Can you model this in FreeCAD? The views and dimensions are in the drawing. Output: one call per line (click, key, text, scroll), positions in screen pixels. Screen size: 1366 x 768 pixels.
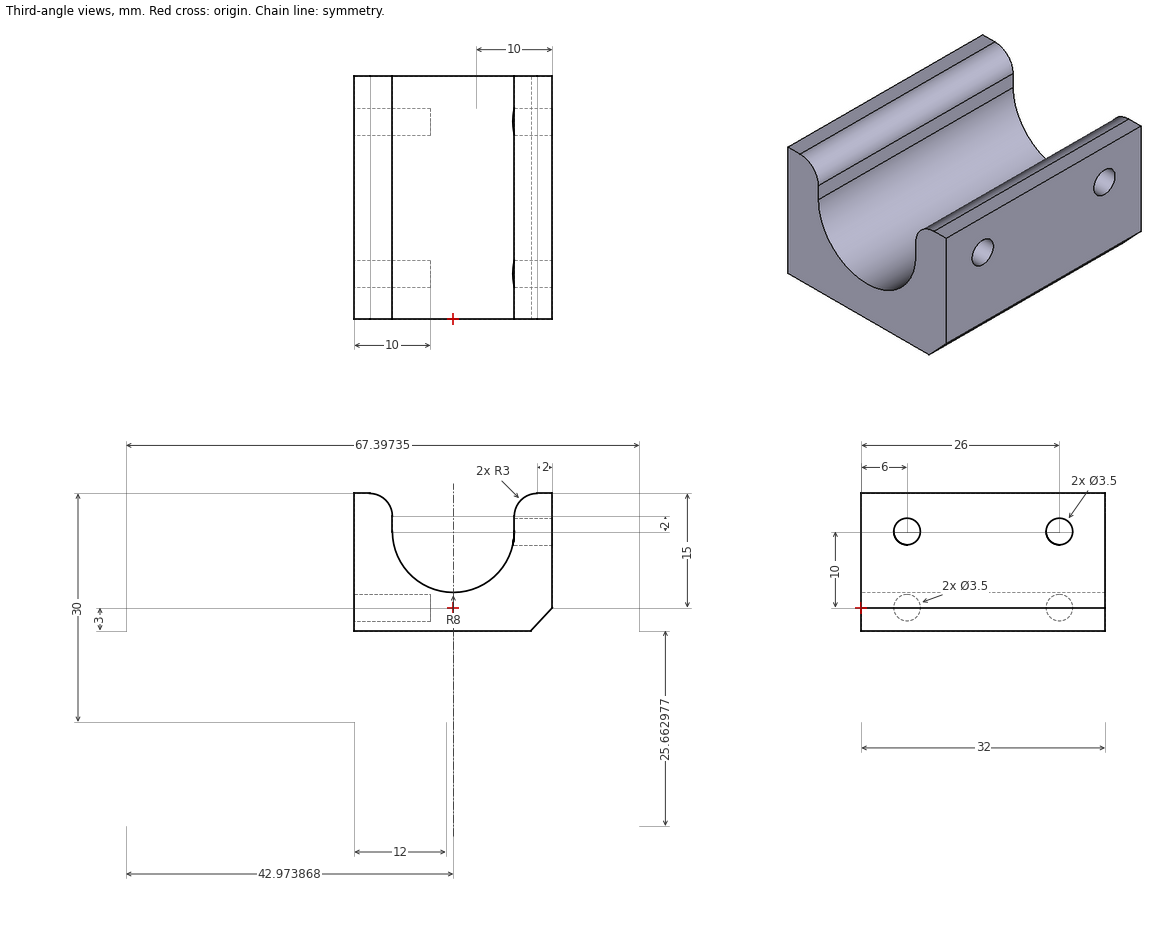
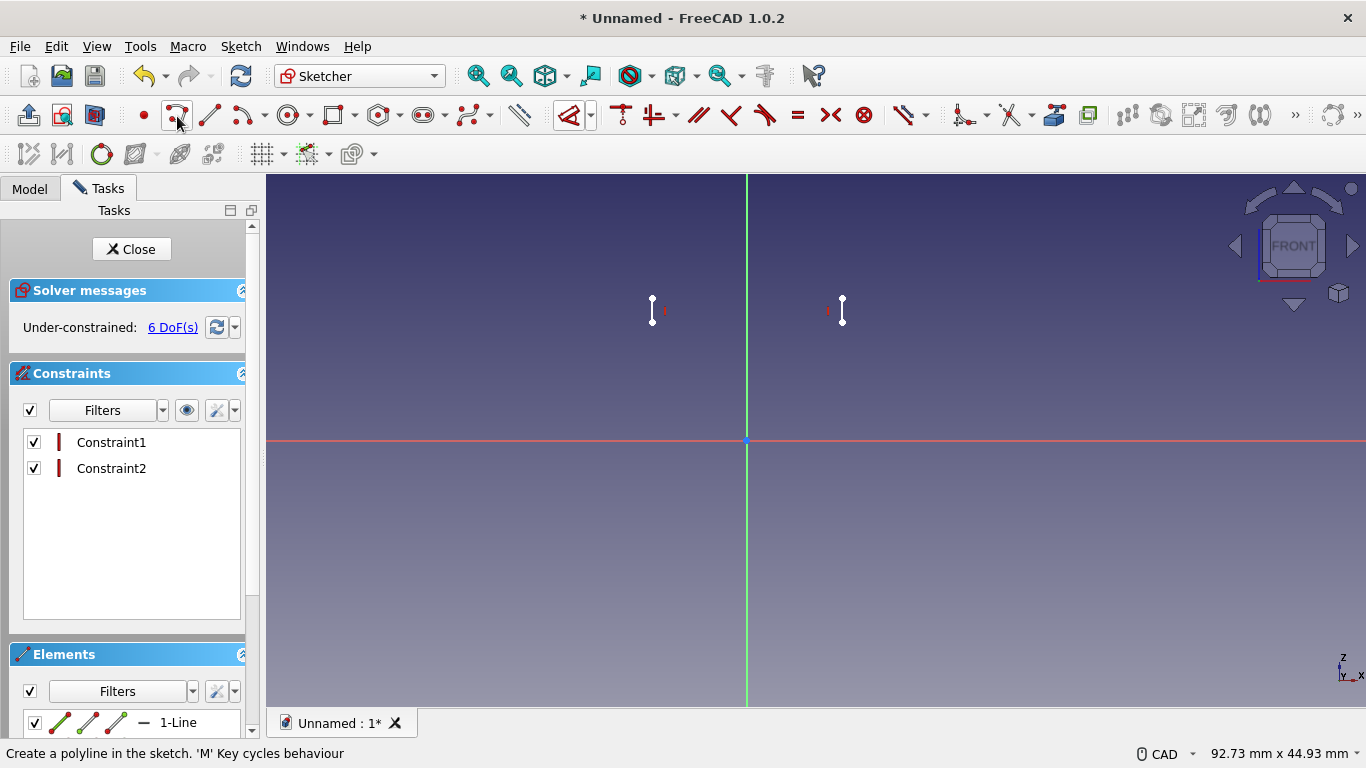
click(877, 263)
click(901, 263)
click(901, 440)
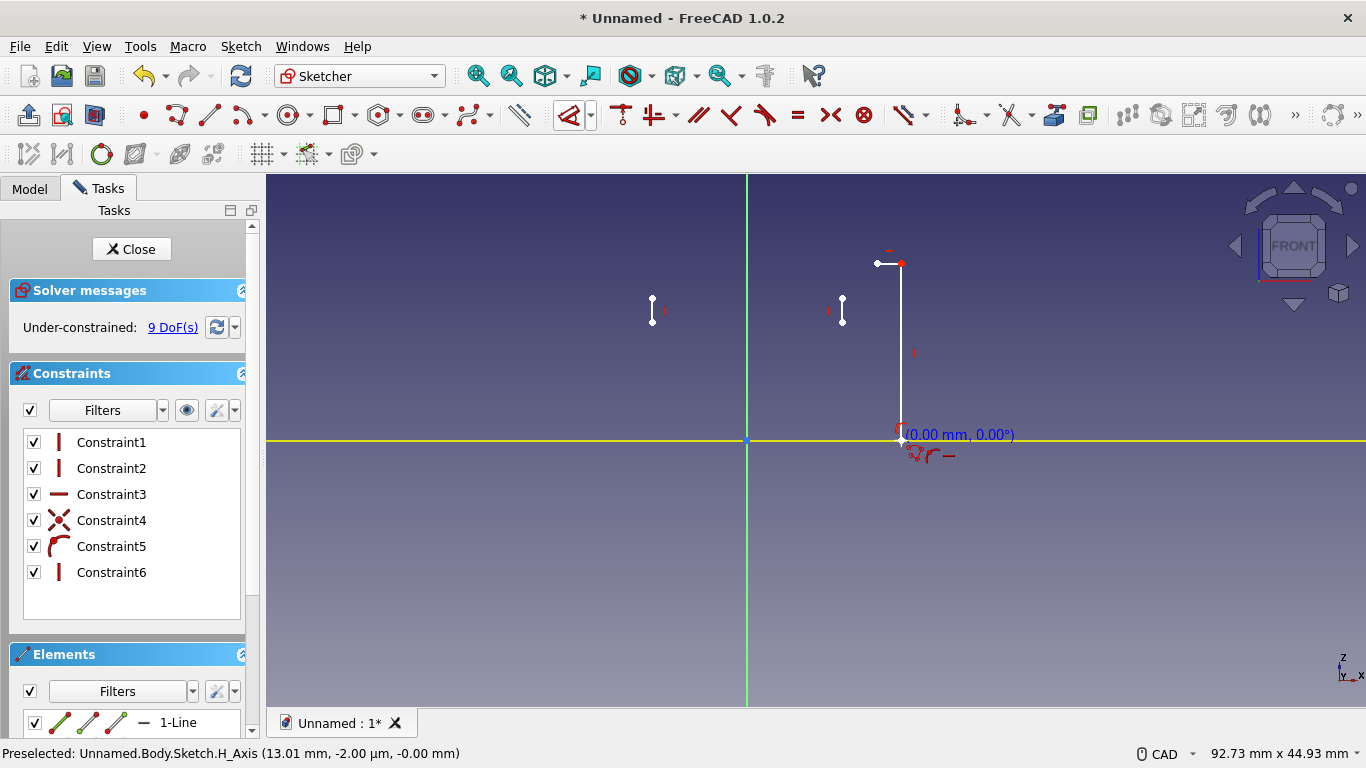
scroll(735, 618, up, 2)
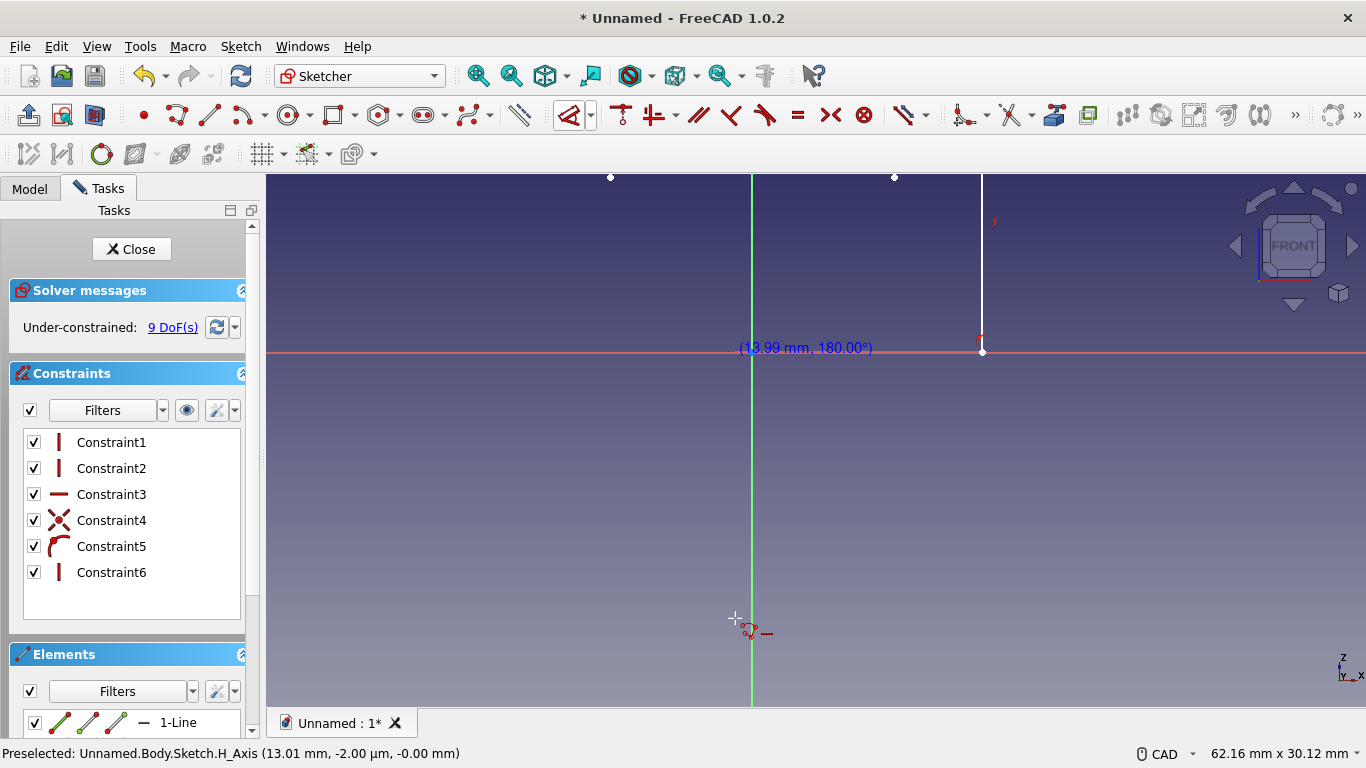
click(735, 618)
click(522, 618)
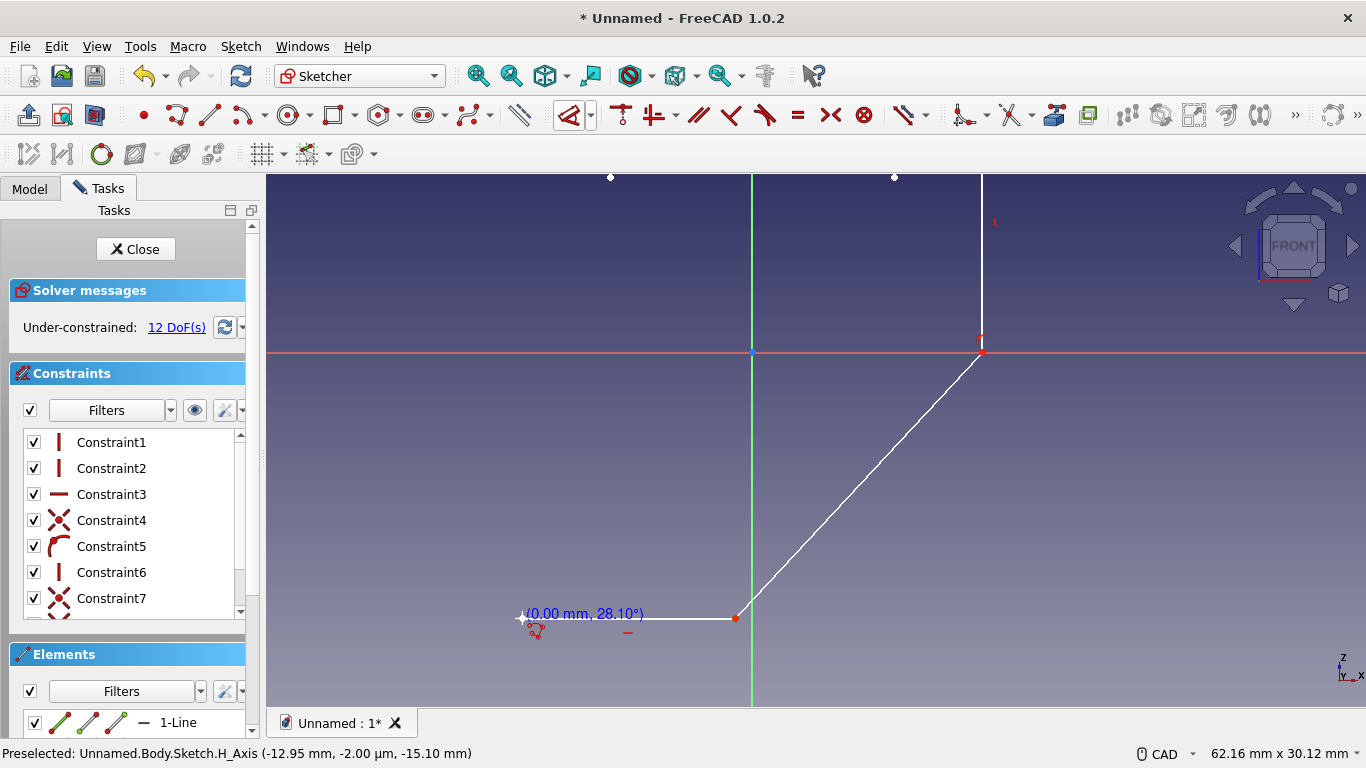
scroll(738, 619, down, 2)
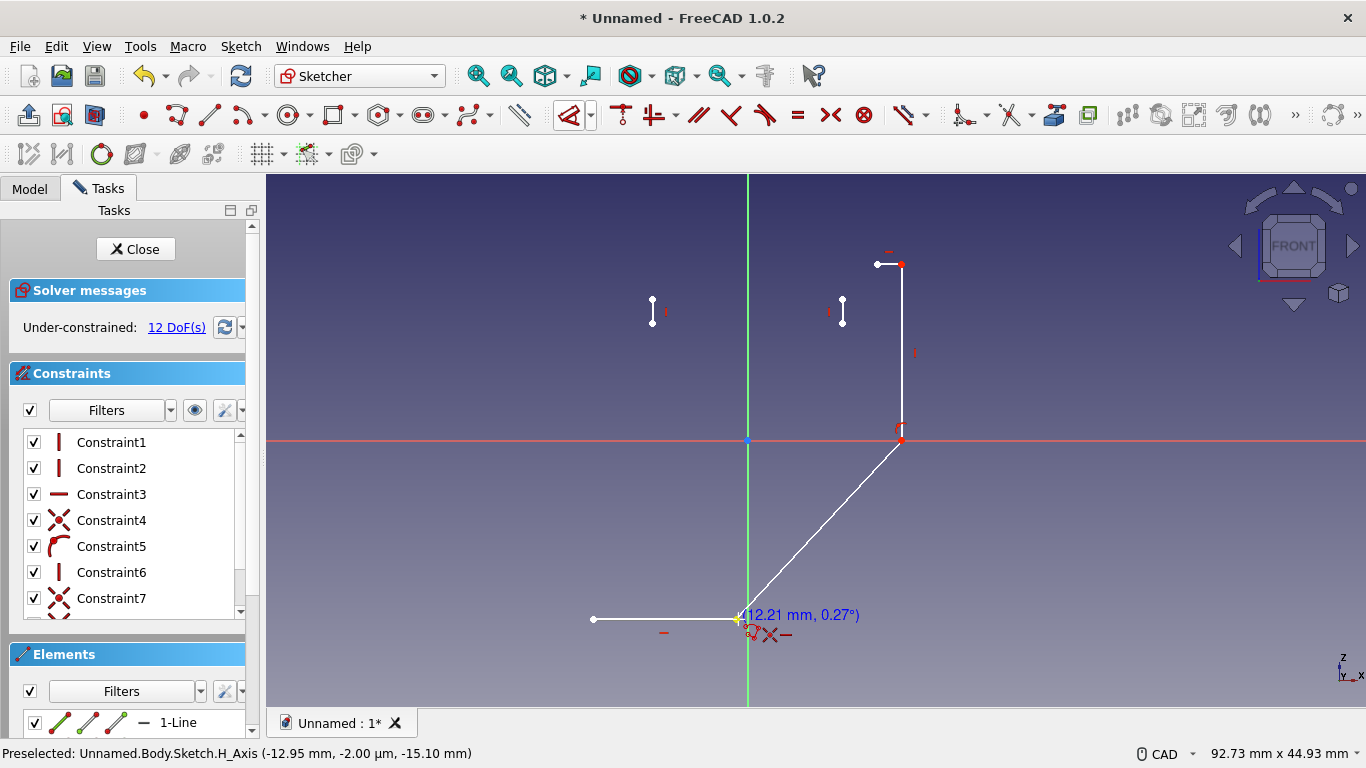
click(593, 263)
click(617, 263)
right_click(617, 263)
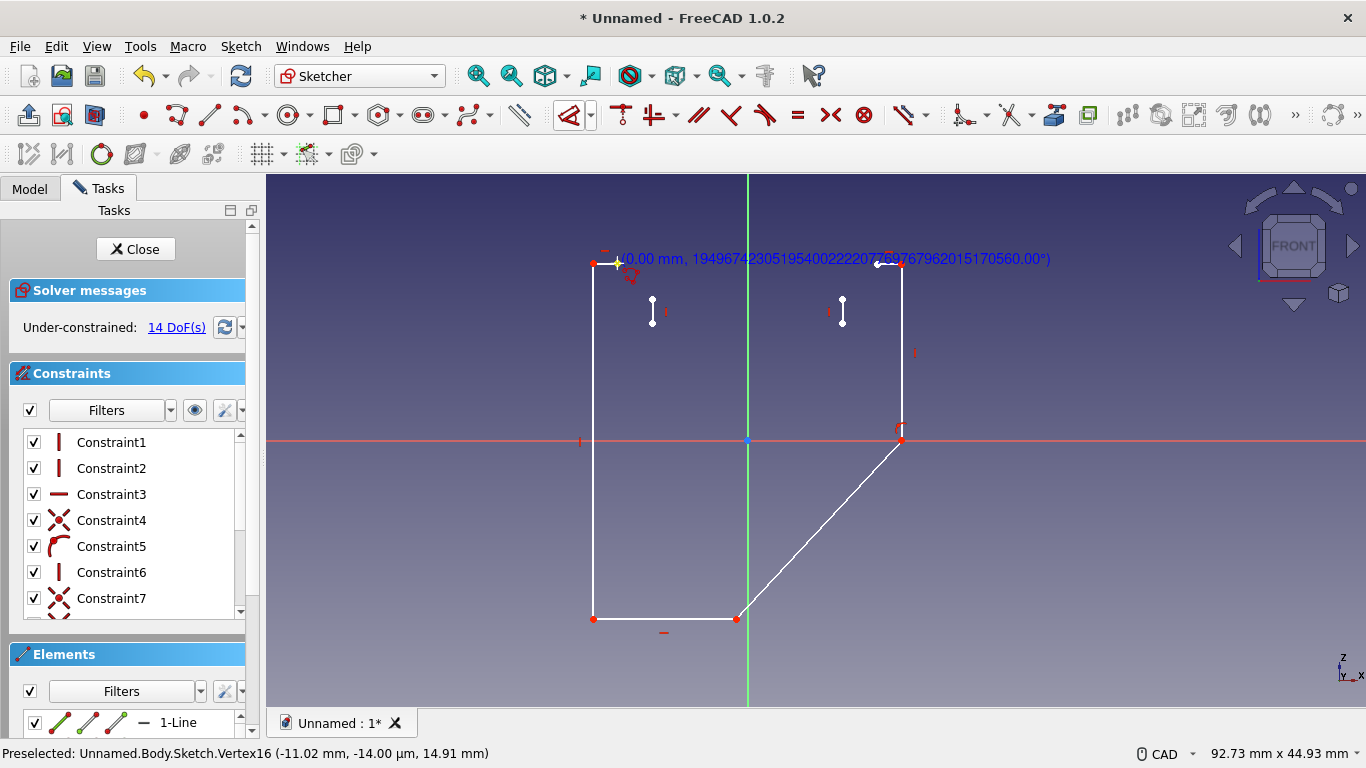
key(g)
key(3)
key(a)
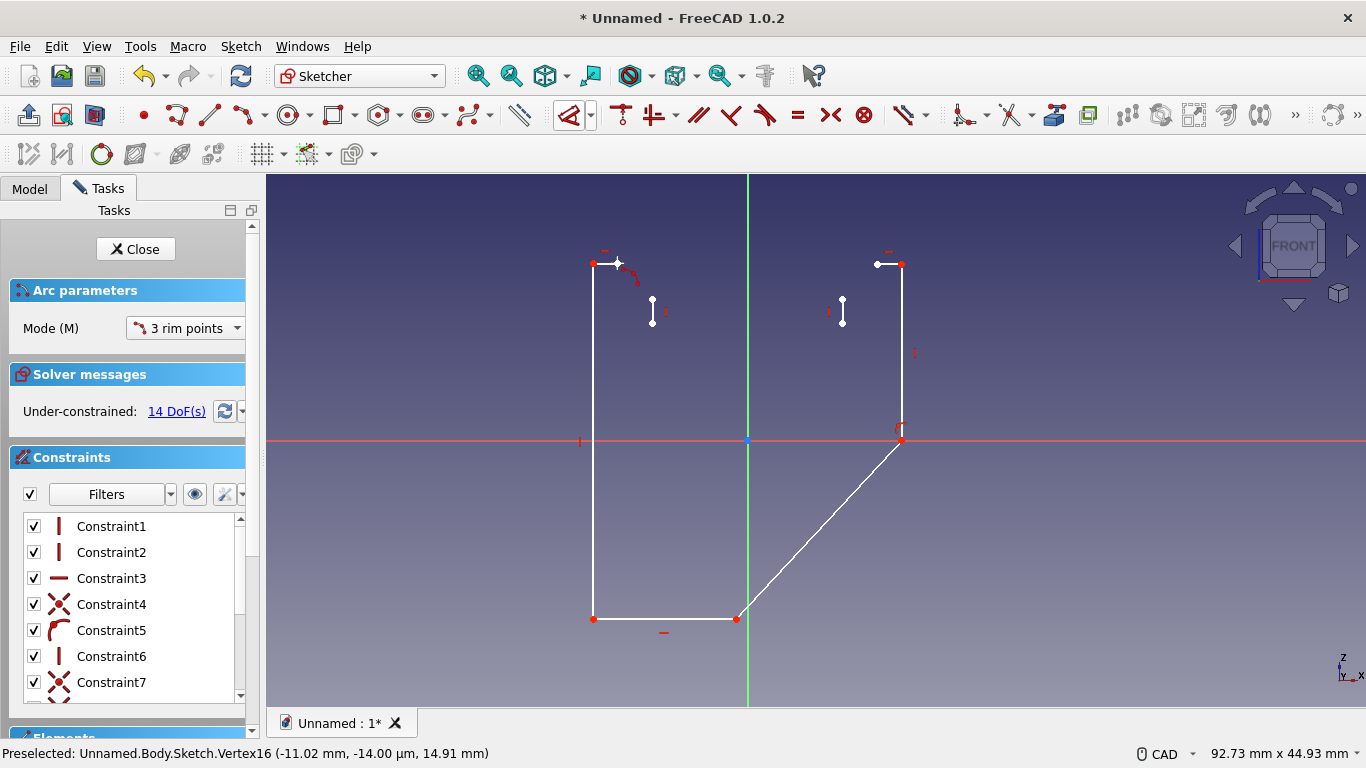
scroll(653, 322, up, 2)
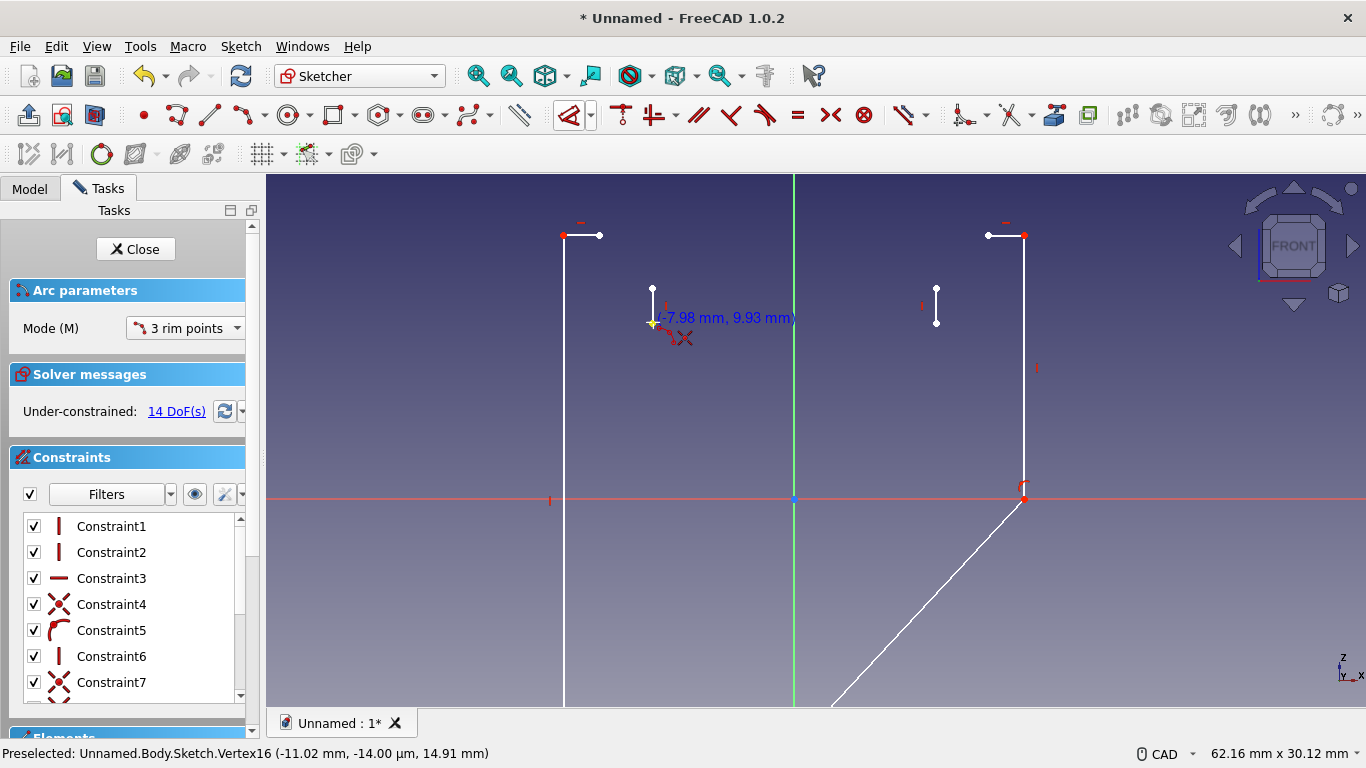
click(653, 324)
click(936, 324)
click(750, 457)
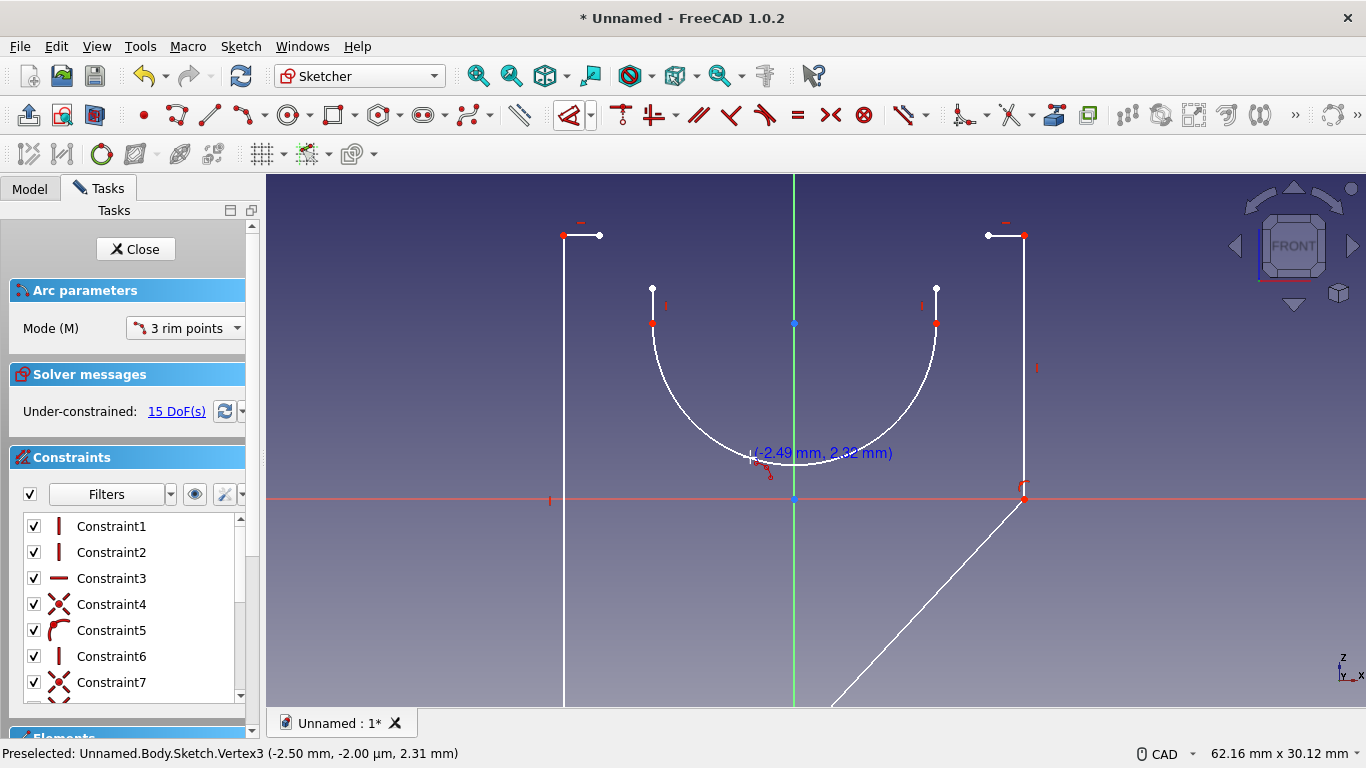
click(936, 288)
click(988, 236)
click(951, 249)